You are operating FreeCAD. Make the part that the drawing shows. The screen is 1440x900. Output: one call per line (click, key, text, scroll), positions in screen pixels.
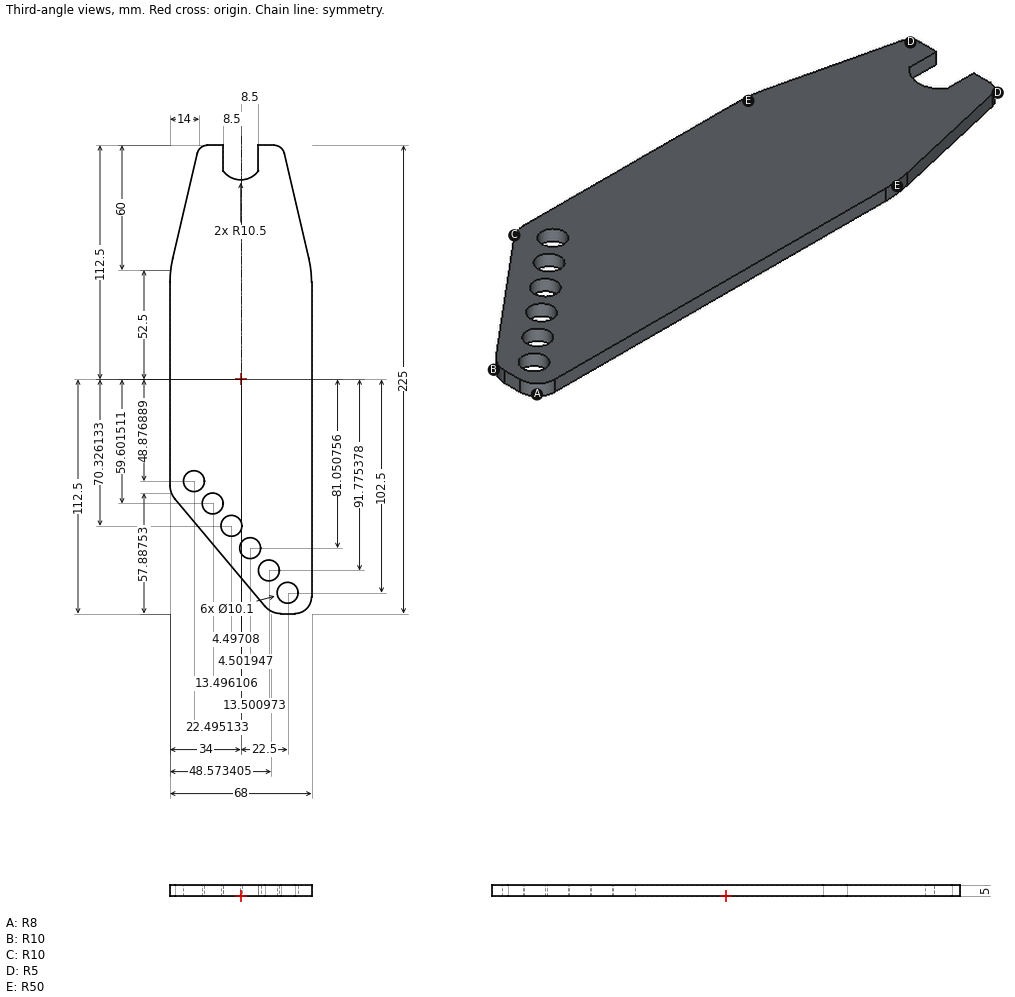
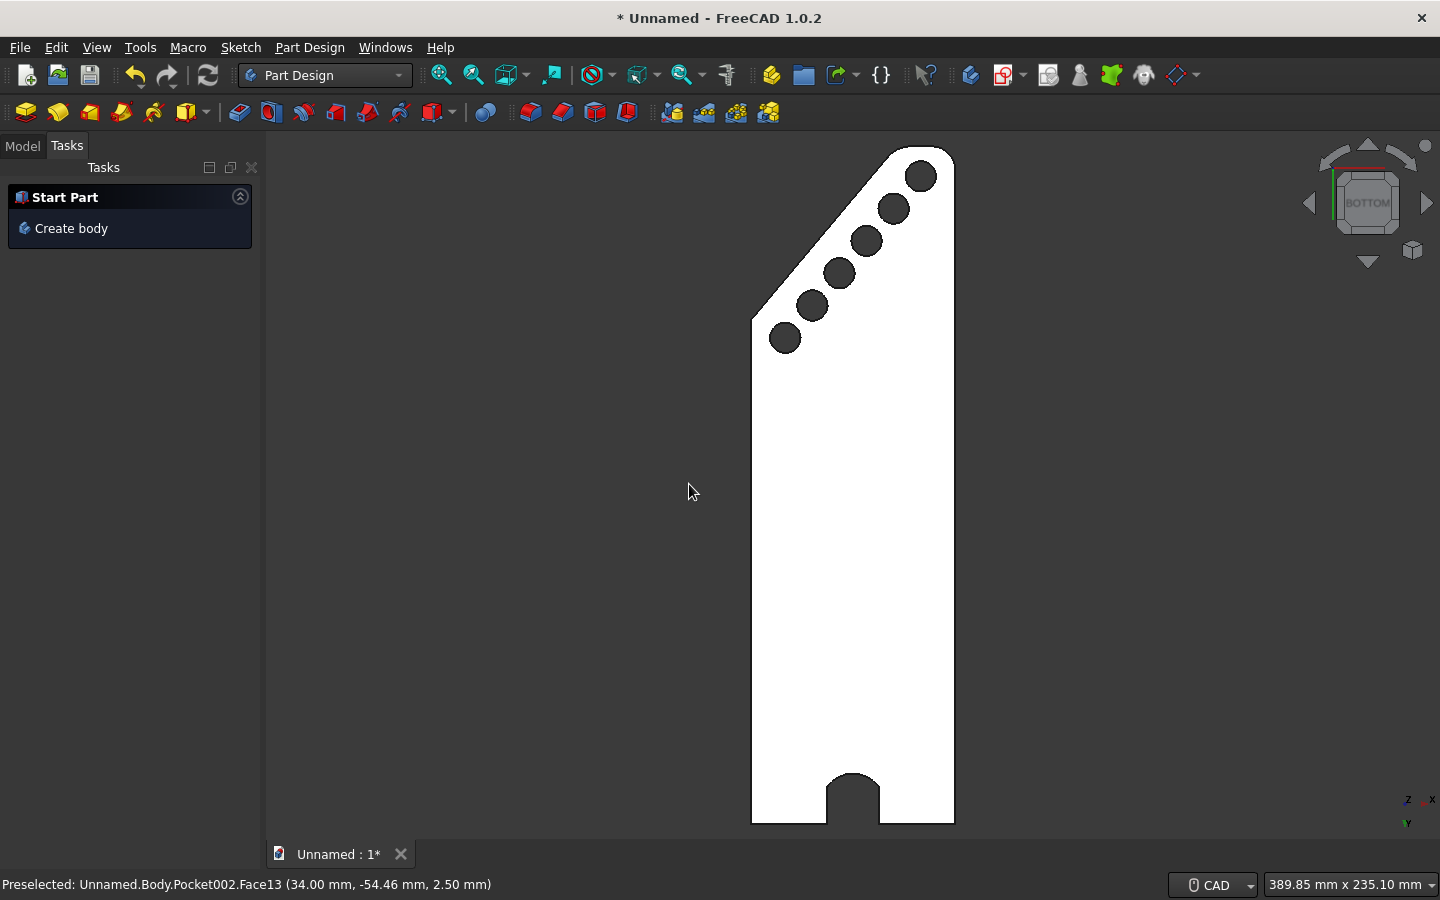
scroll(751, 320, up, 5)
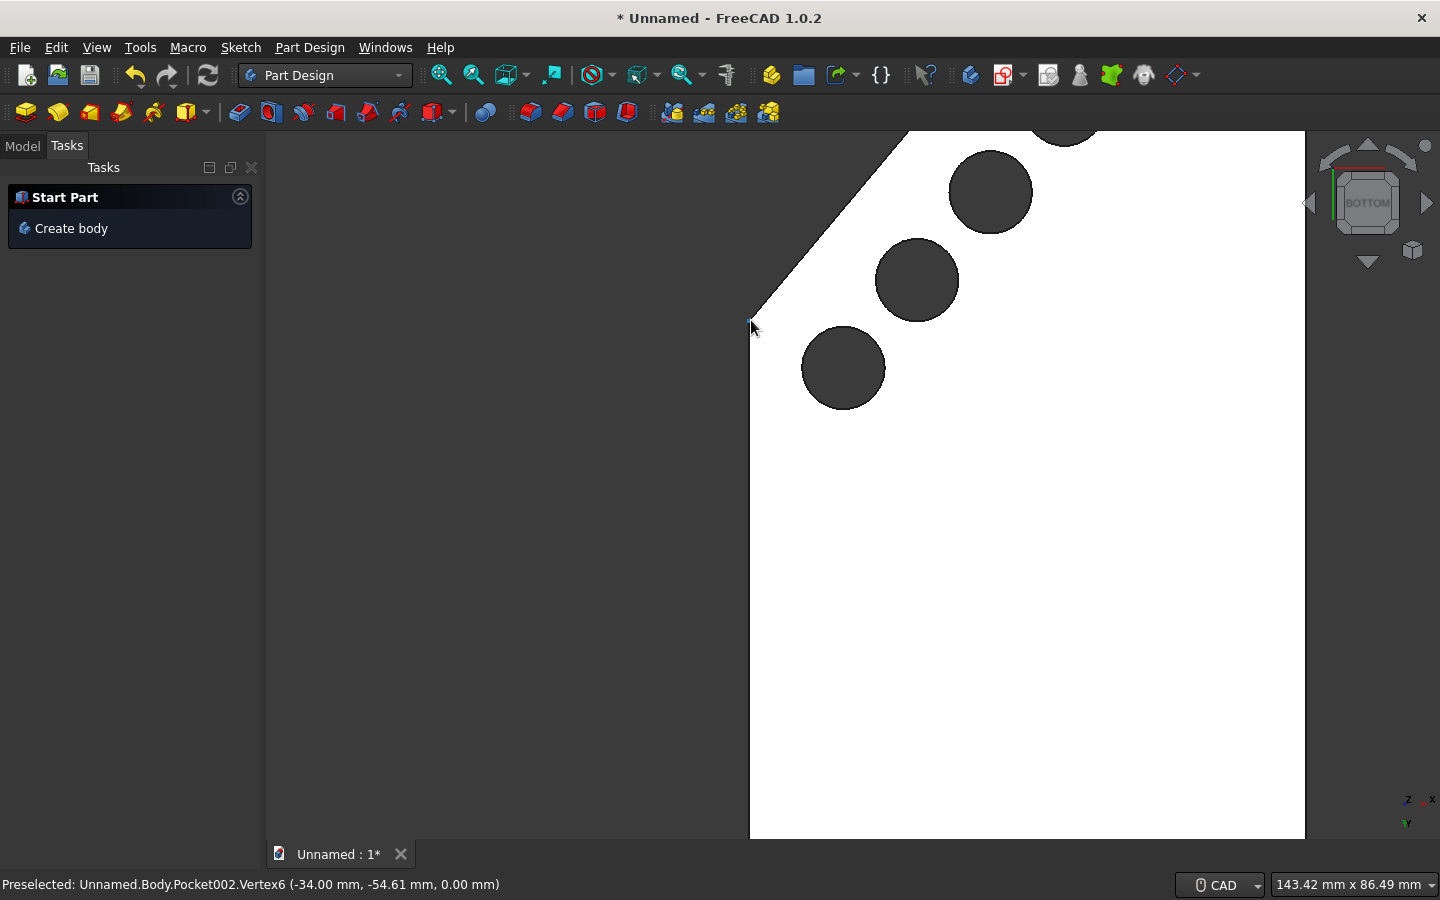
click(442, 76)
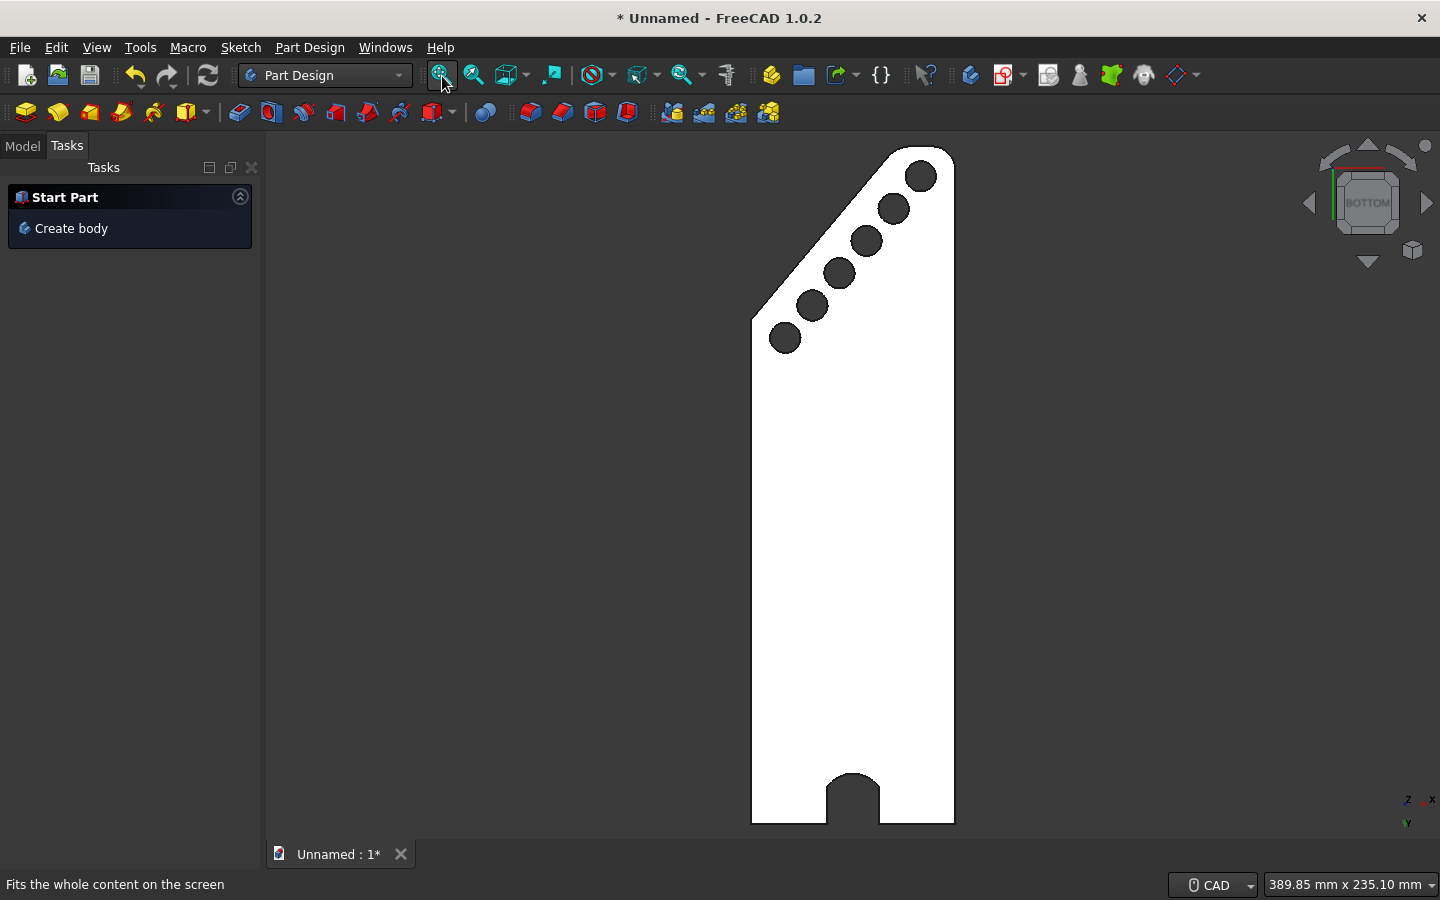
key(4)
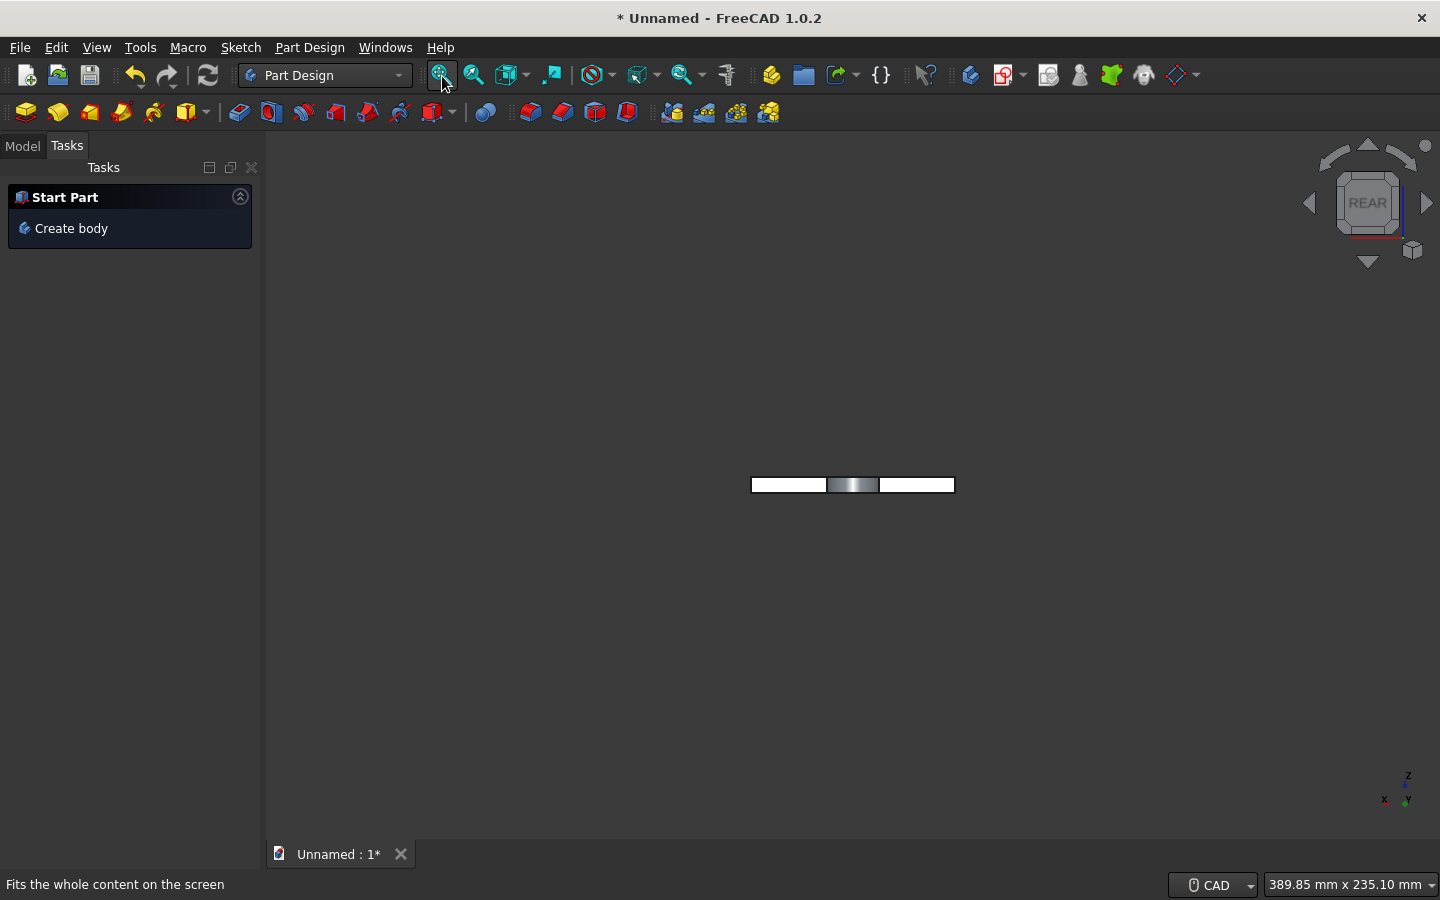
key(v)
key(f)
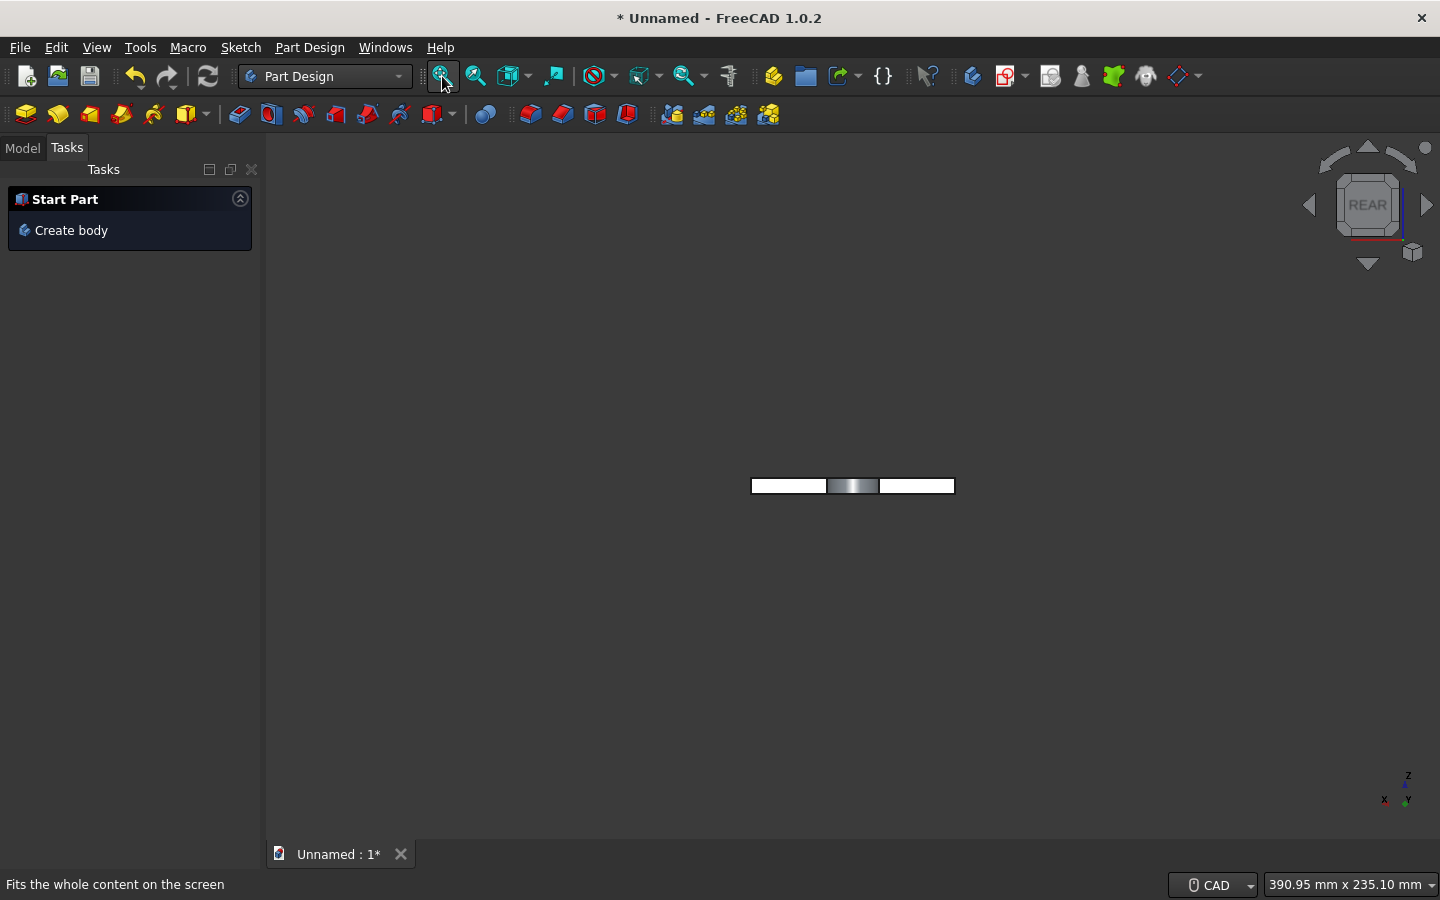
scroll(955, 485, up, 5)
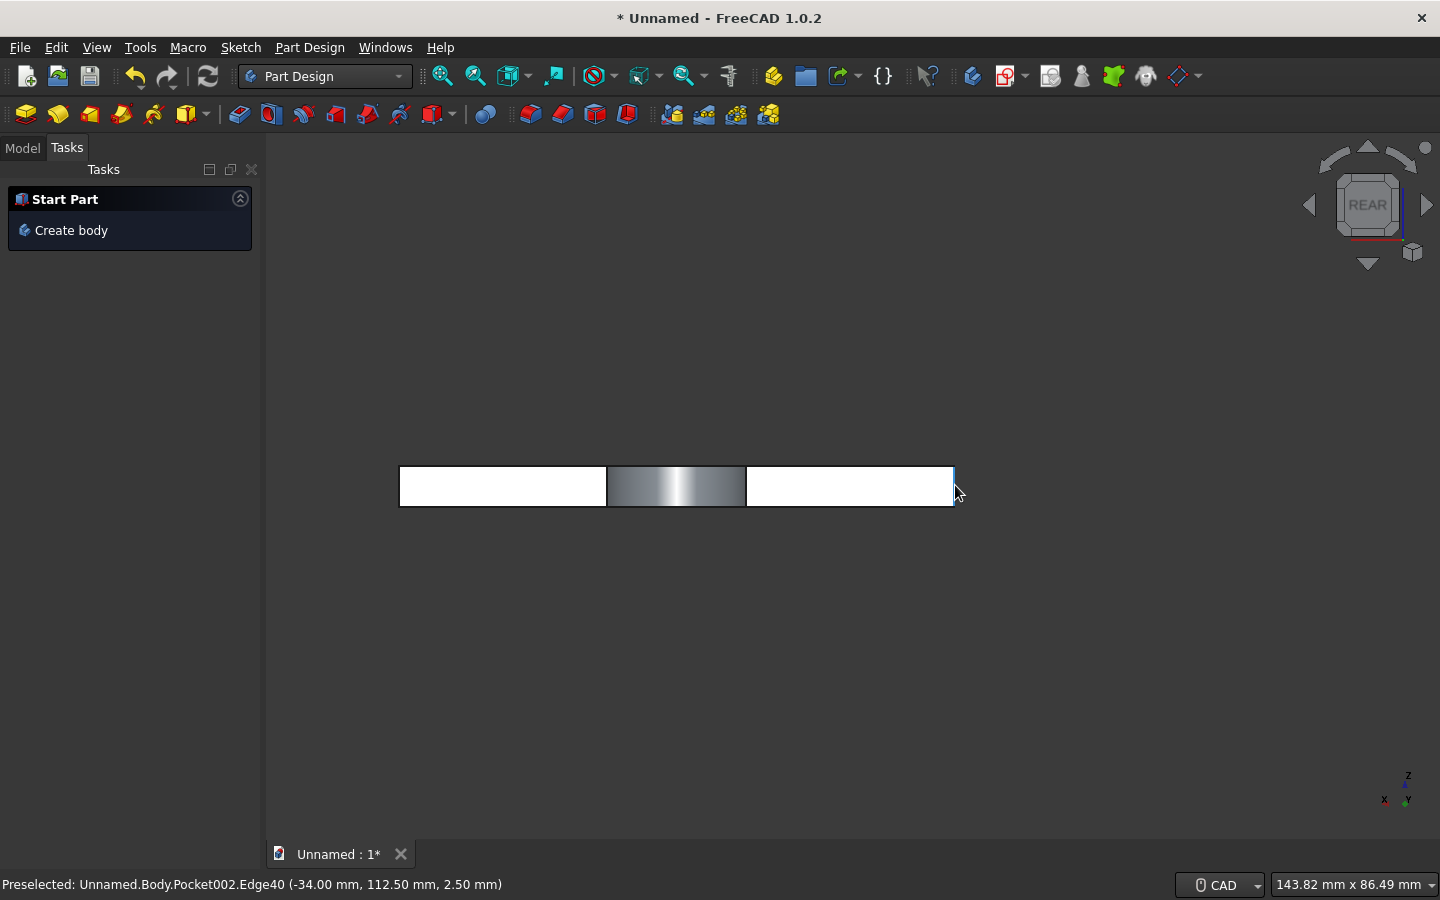
key(v)
key(f)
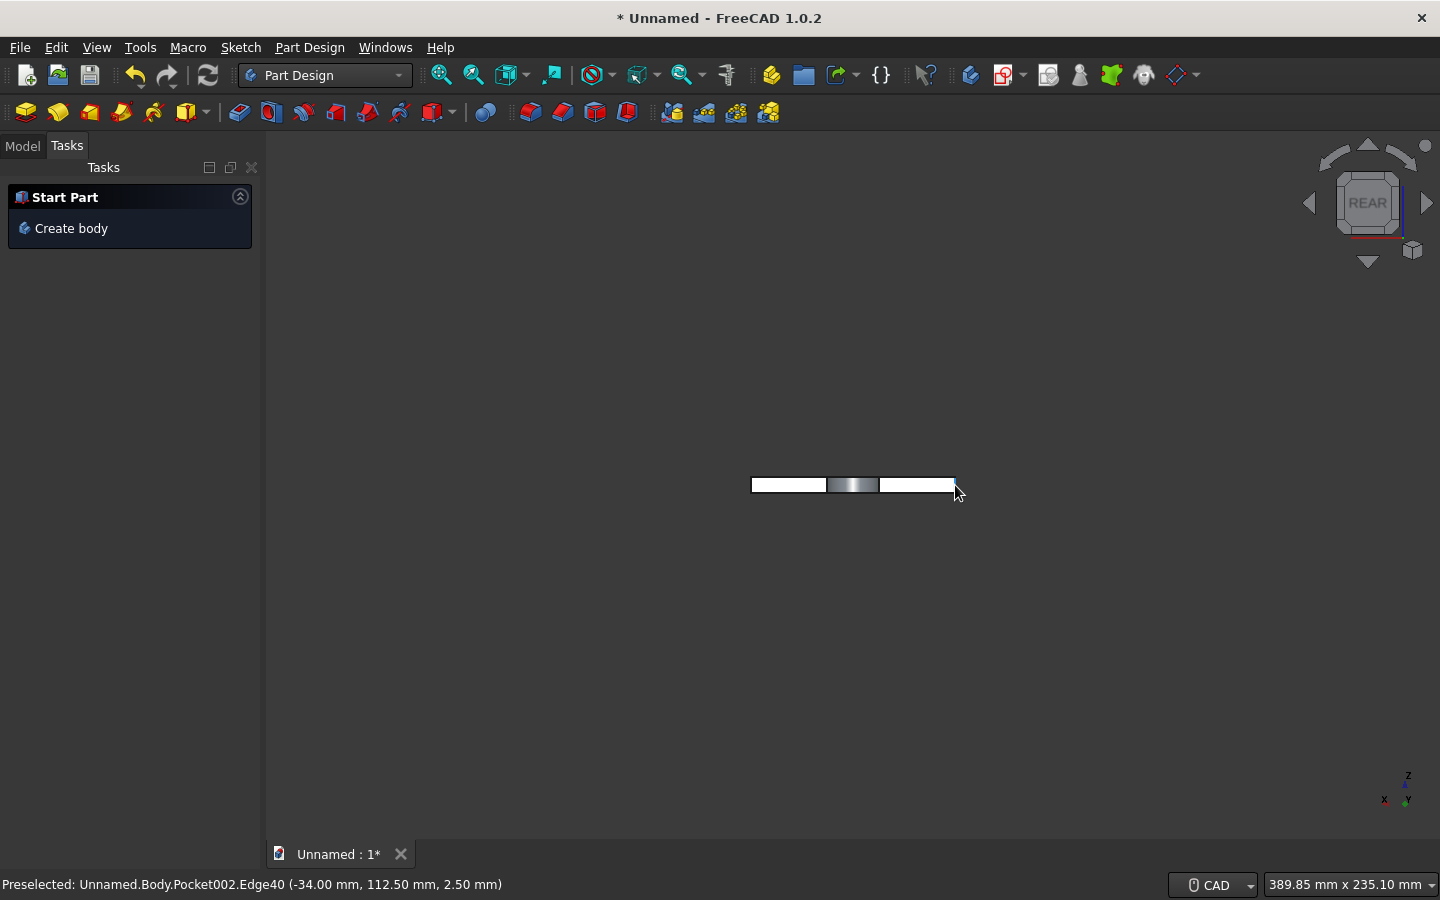
key(6)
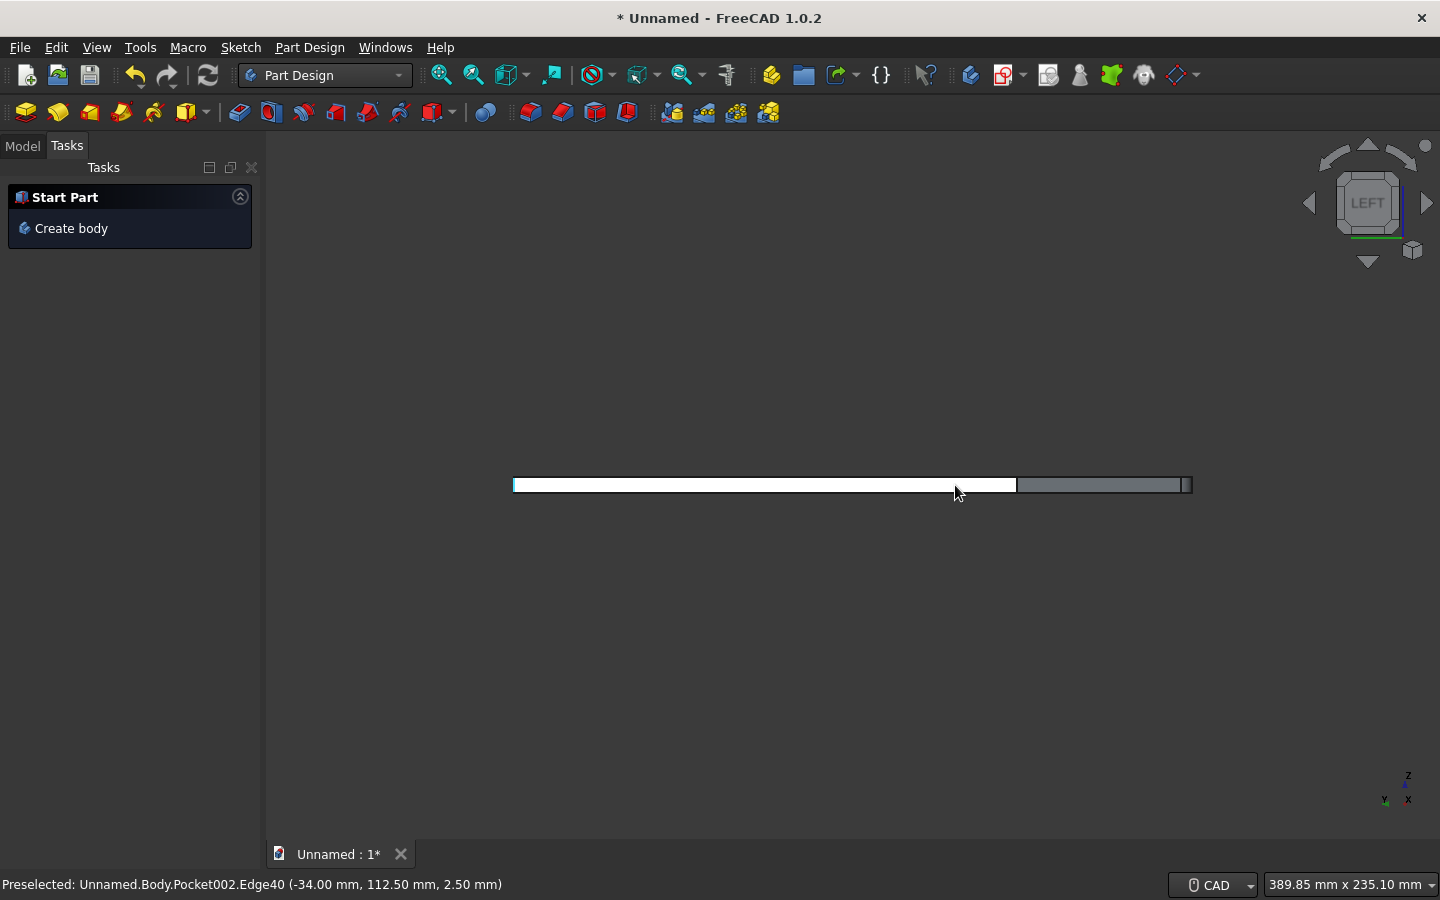
click(1017, 484)